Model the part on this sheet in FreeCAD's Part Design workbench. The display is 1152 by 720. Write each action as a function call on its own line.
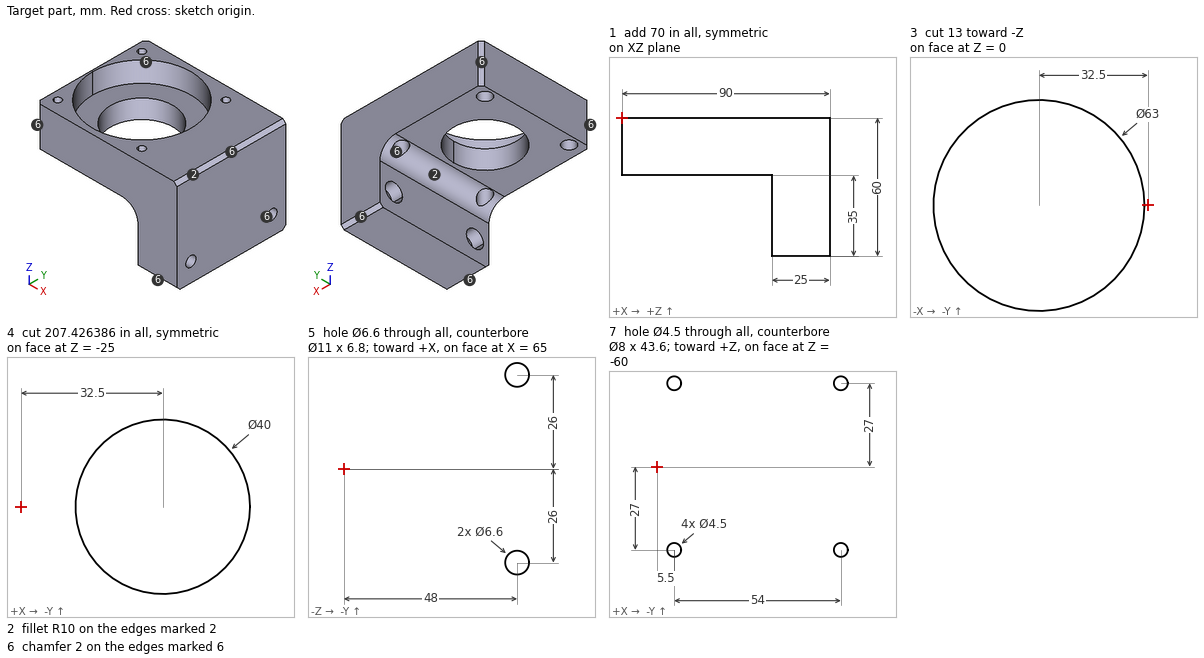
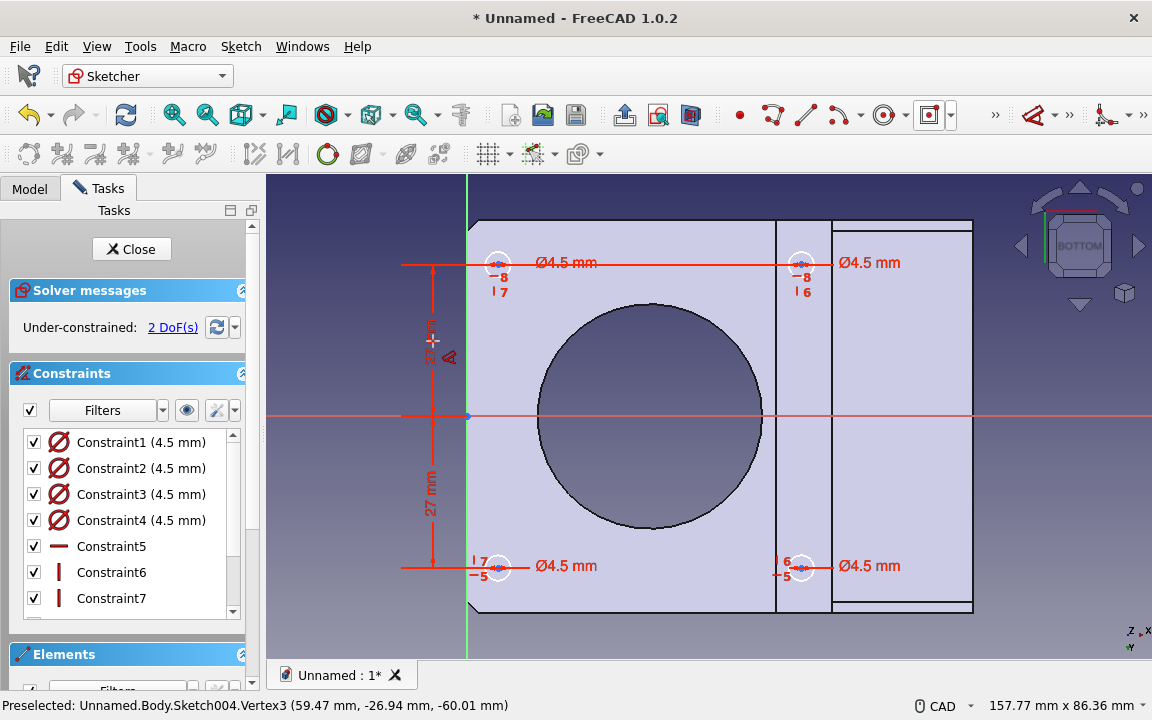
scroll(498, 568, up, 2)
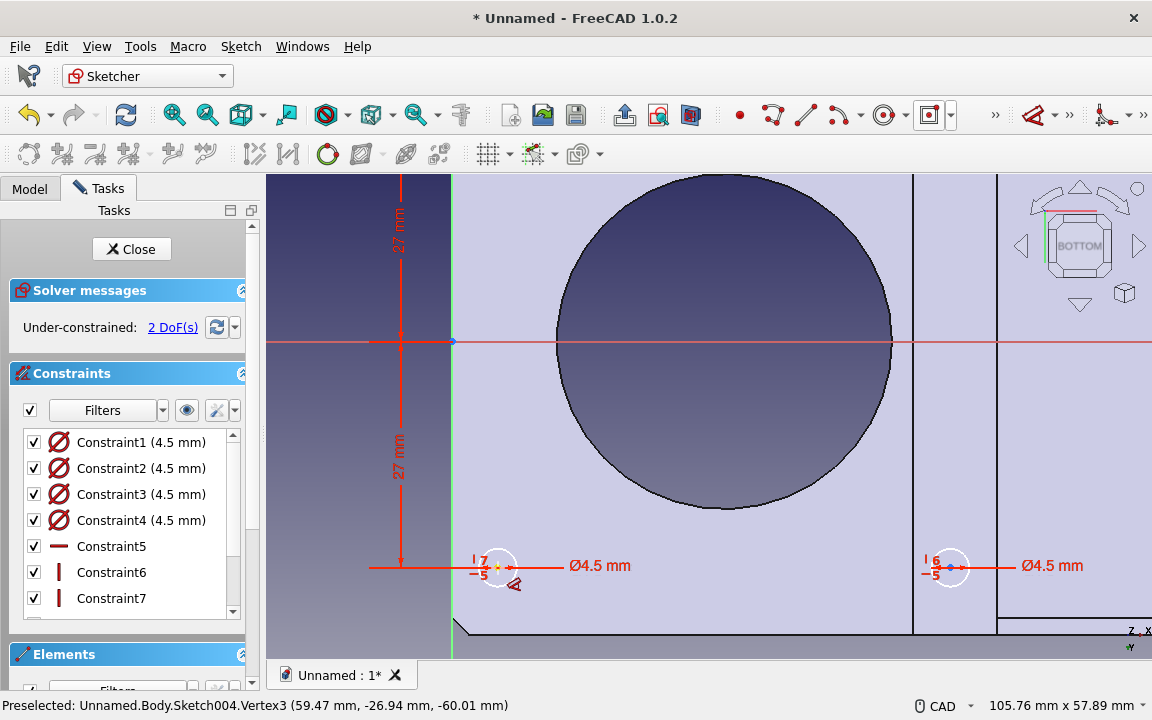
click(498, 568)
click(475, 602)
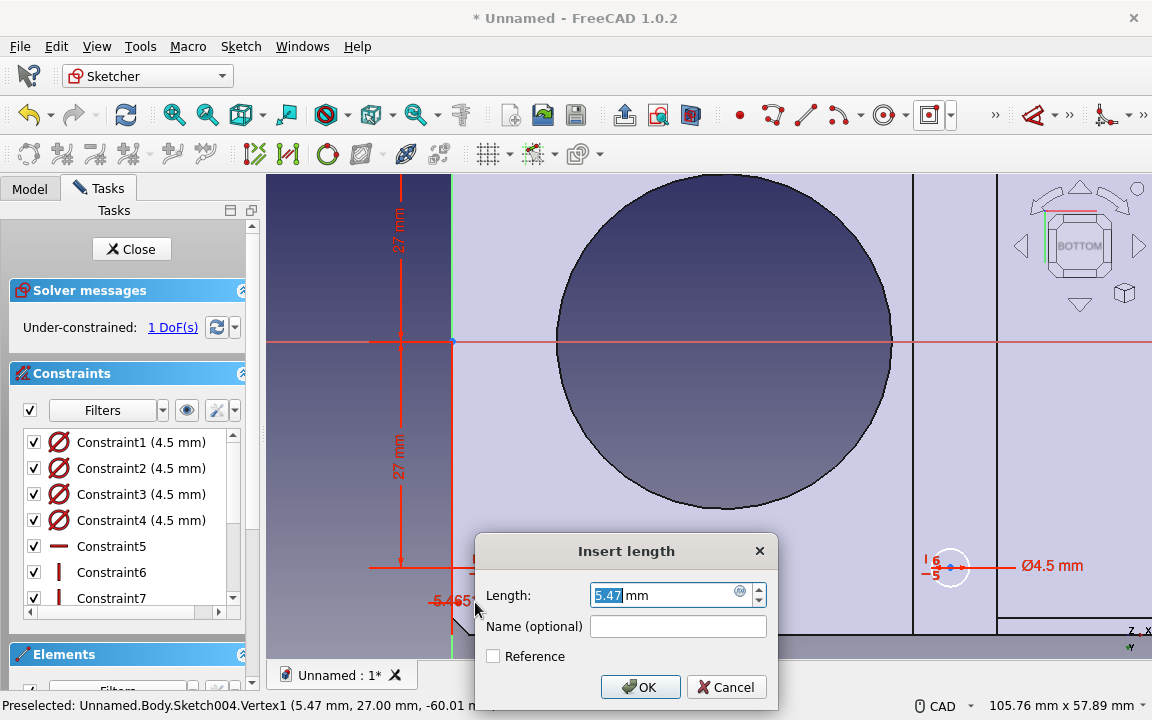
text(5.5)
key(Return)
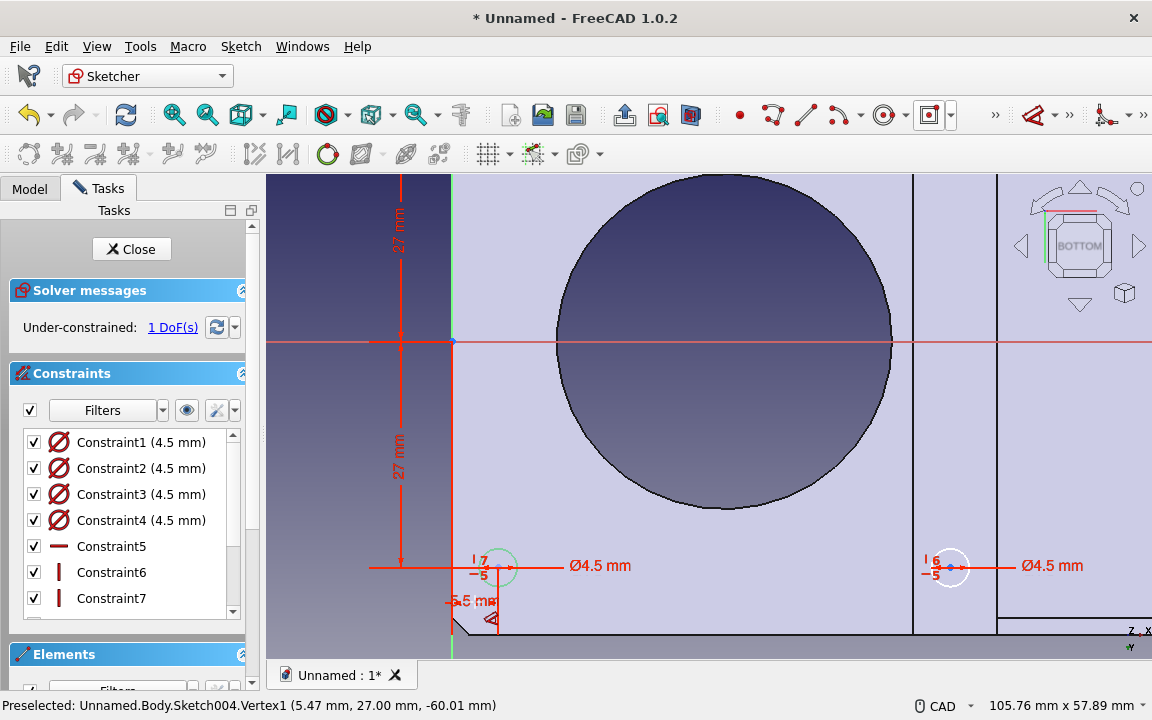
click(498, 568)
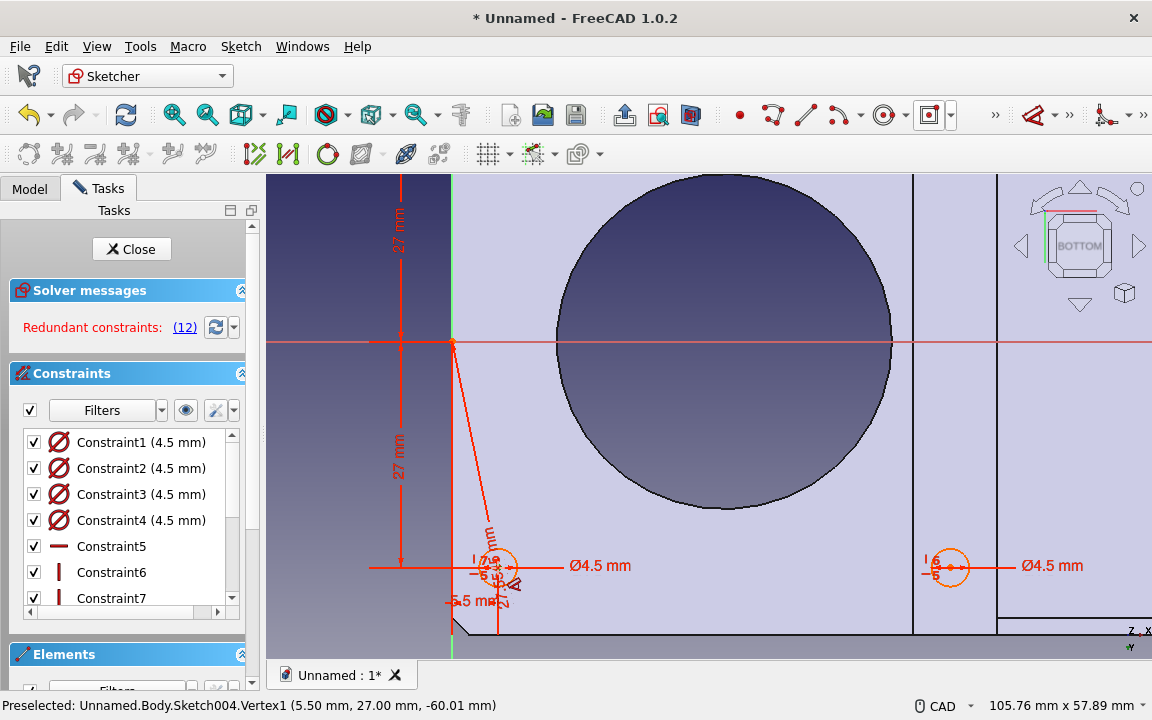
click(950, 568)
click(724, 602)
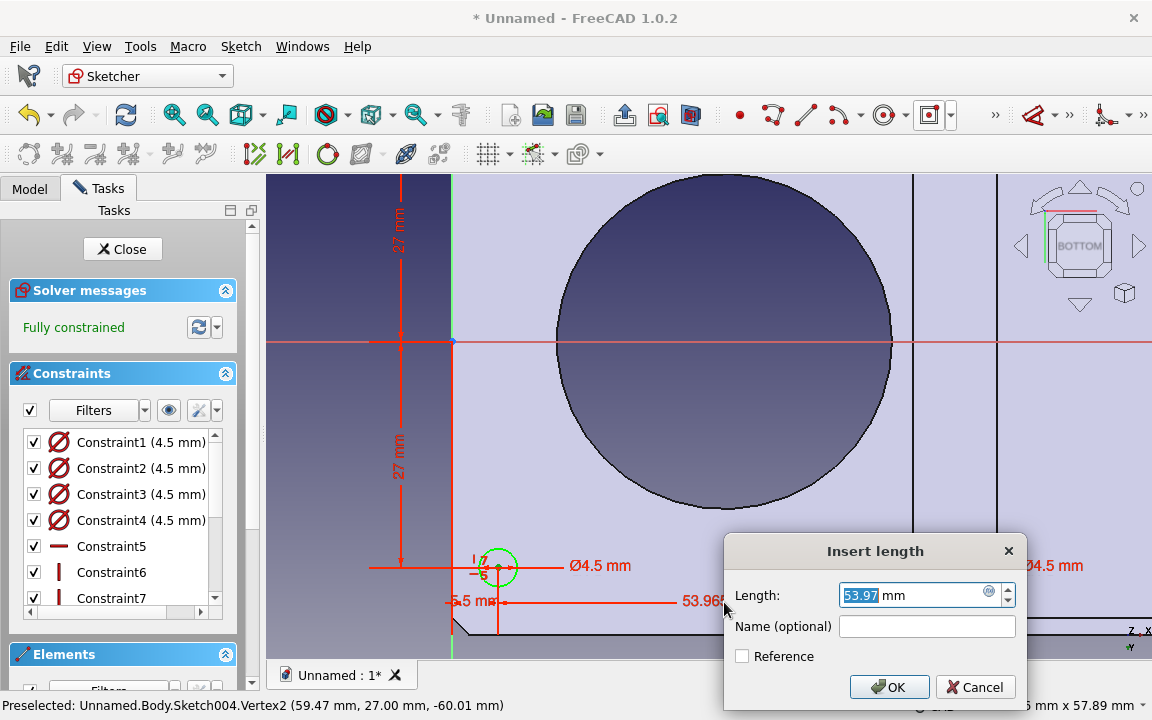
text(54)
key(Return)
key(Escape)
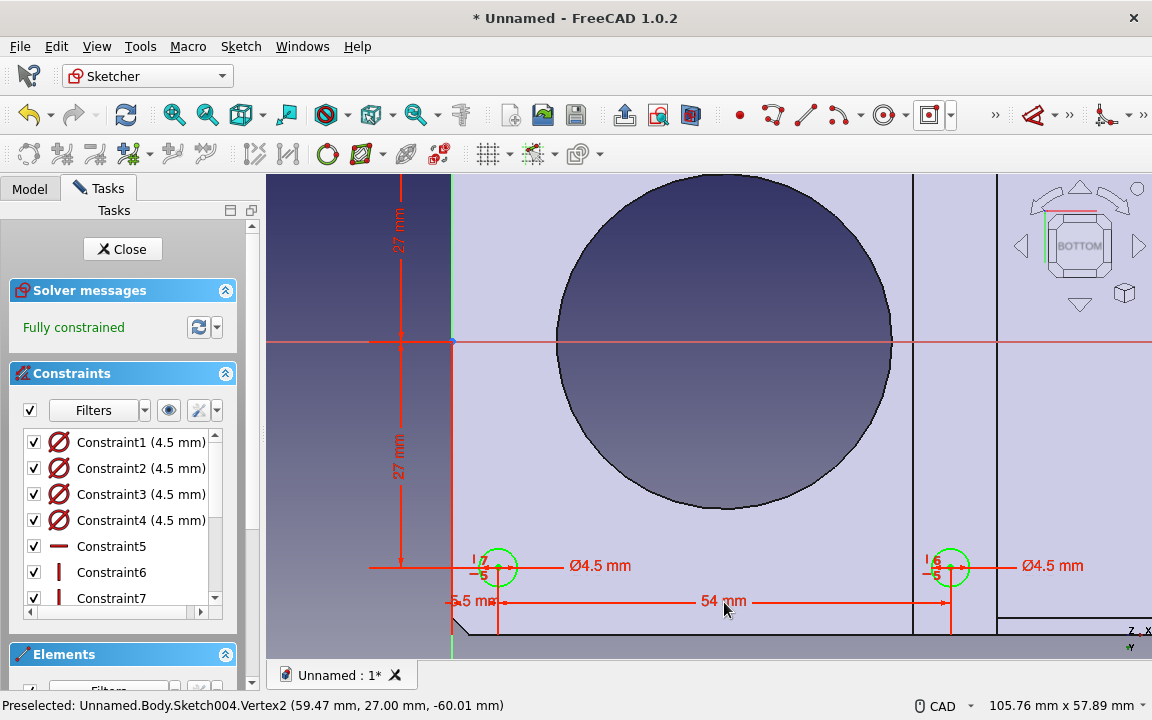
click(123, 249)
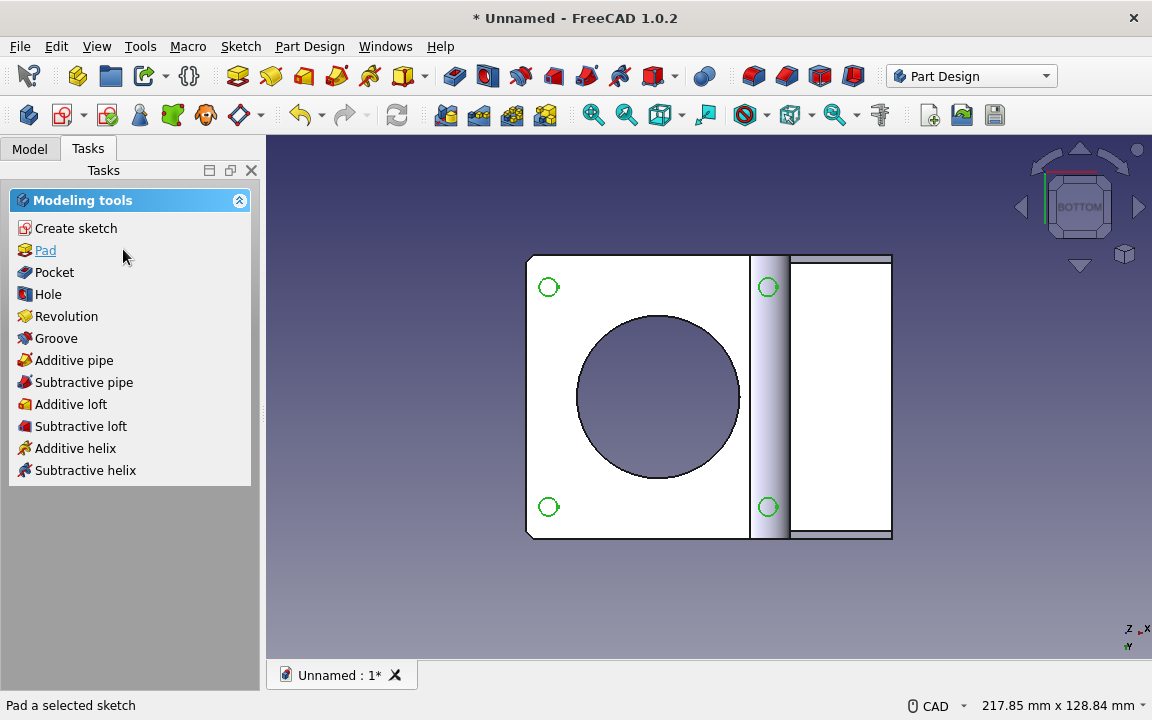
click(488, 76)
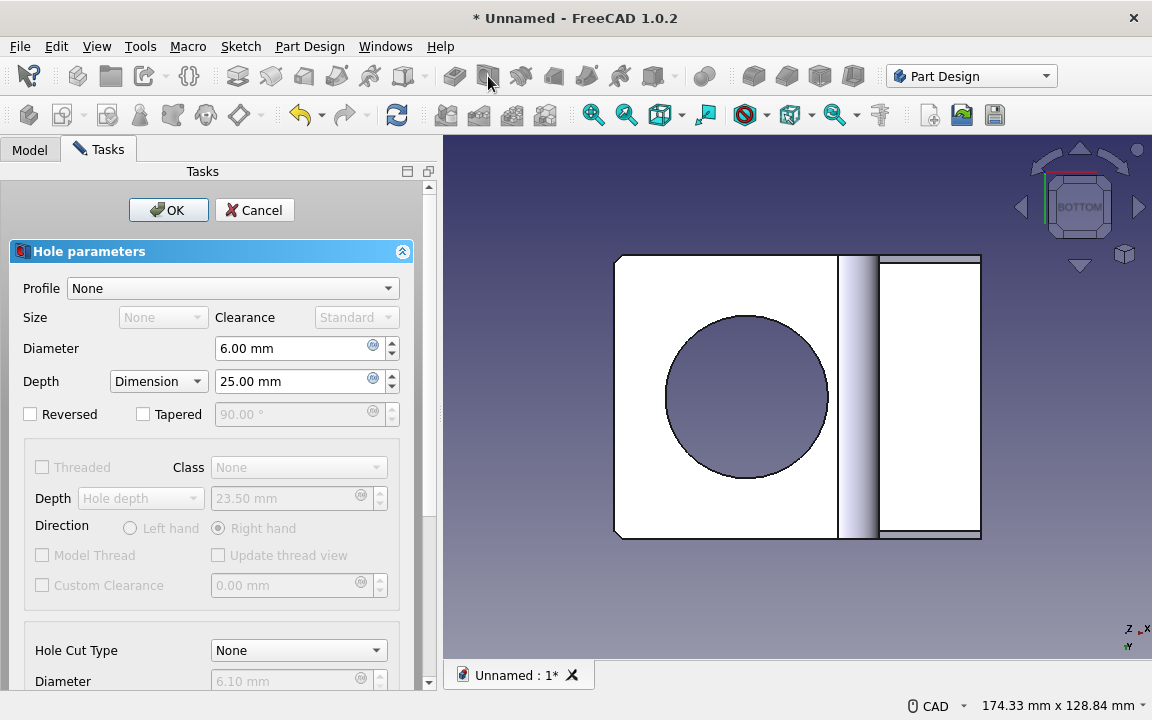
triple_click(300, 348)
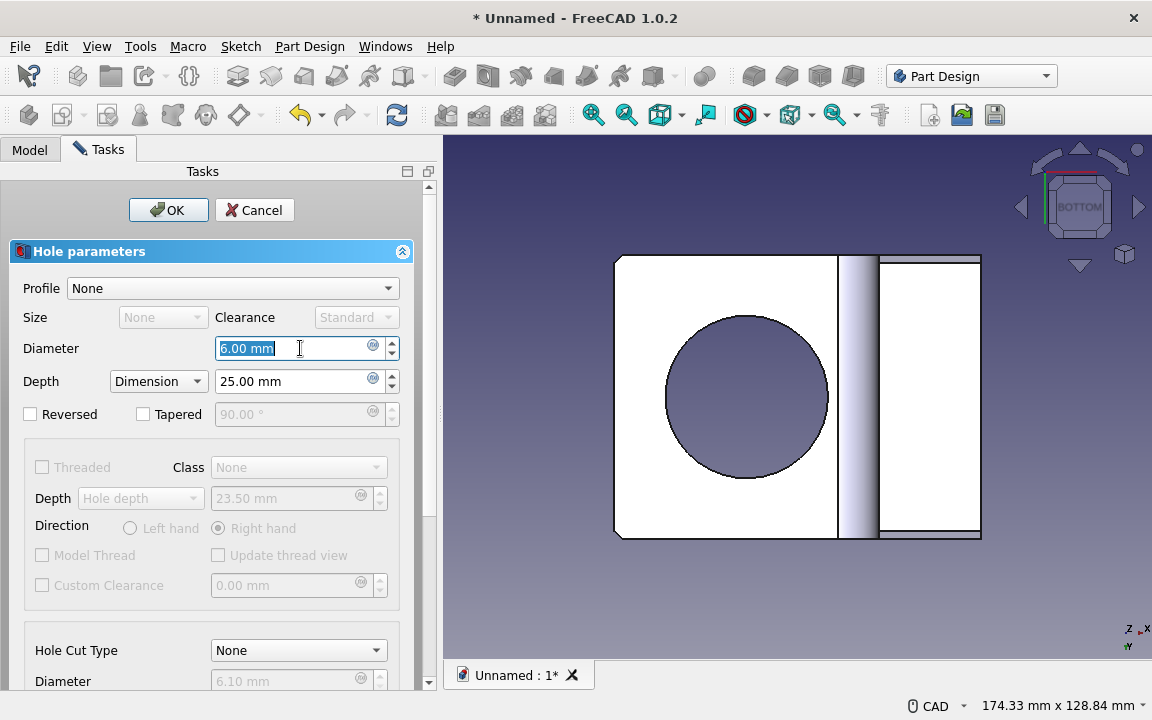
text(4.5)
key(Tab)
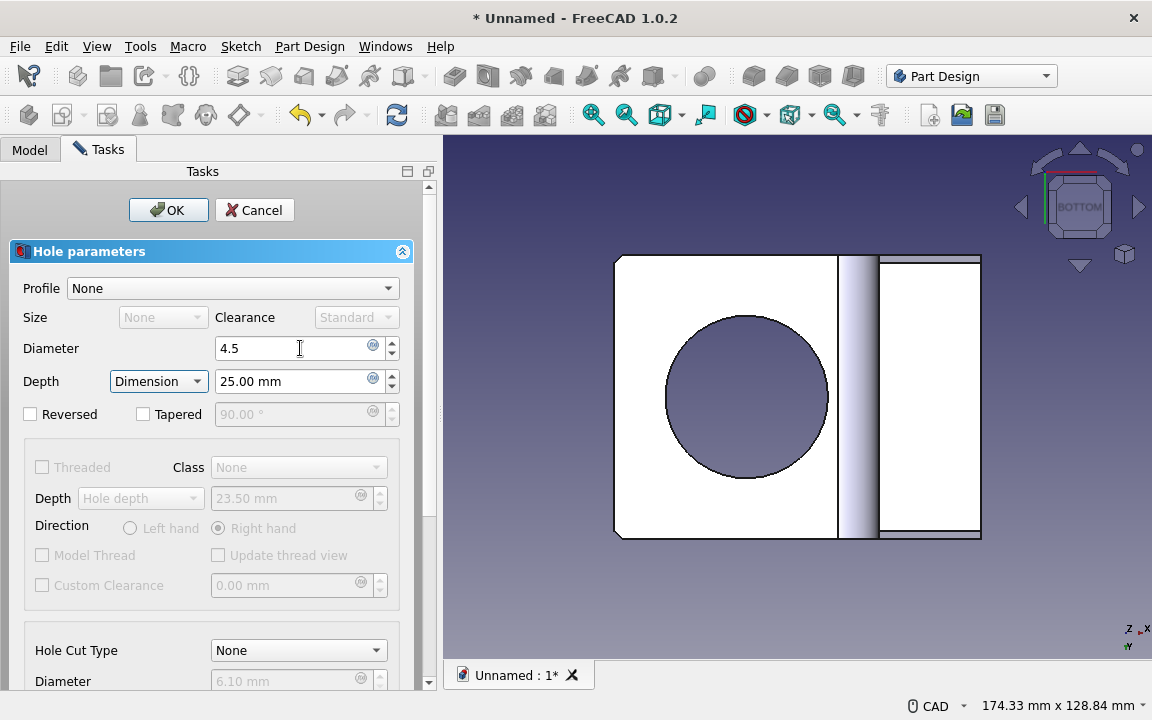
click(160, 382)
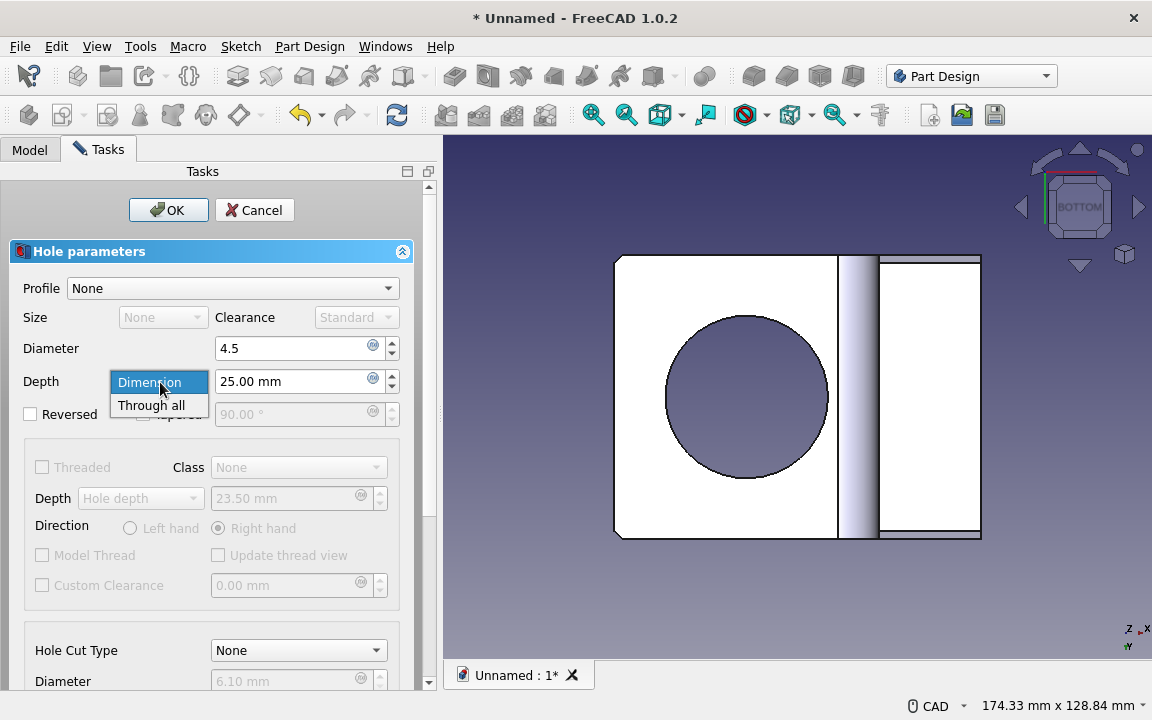
click(158, 406)